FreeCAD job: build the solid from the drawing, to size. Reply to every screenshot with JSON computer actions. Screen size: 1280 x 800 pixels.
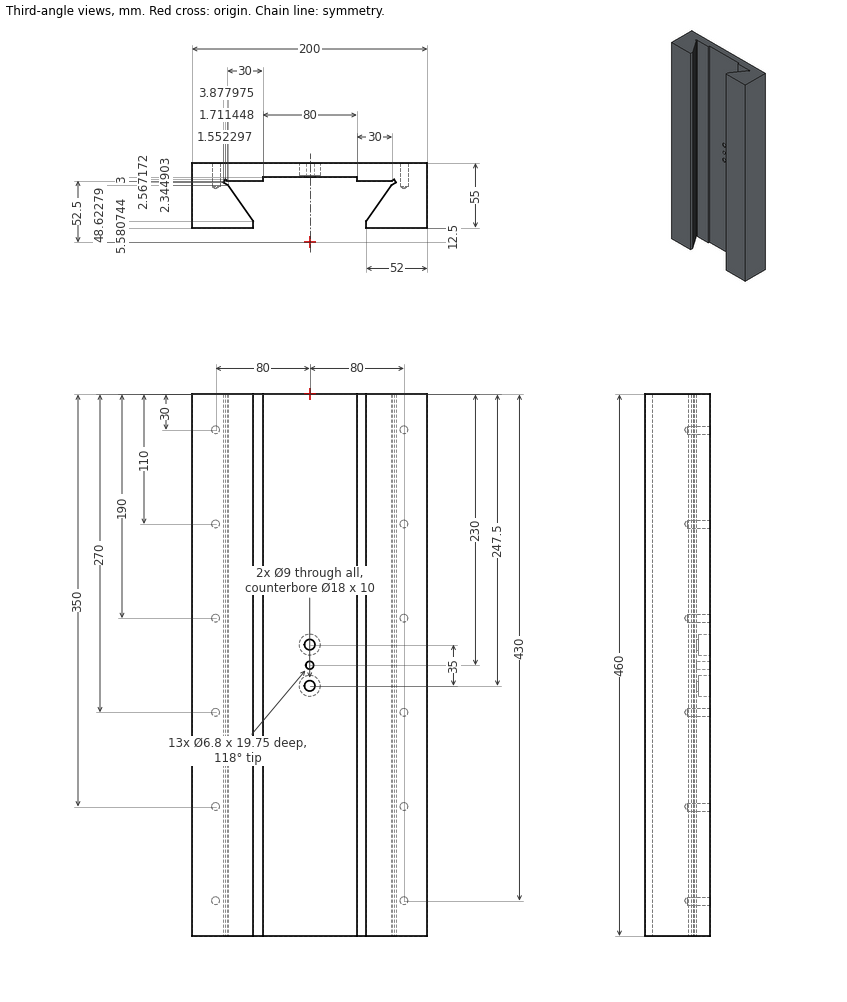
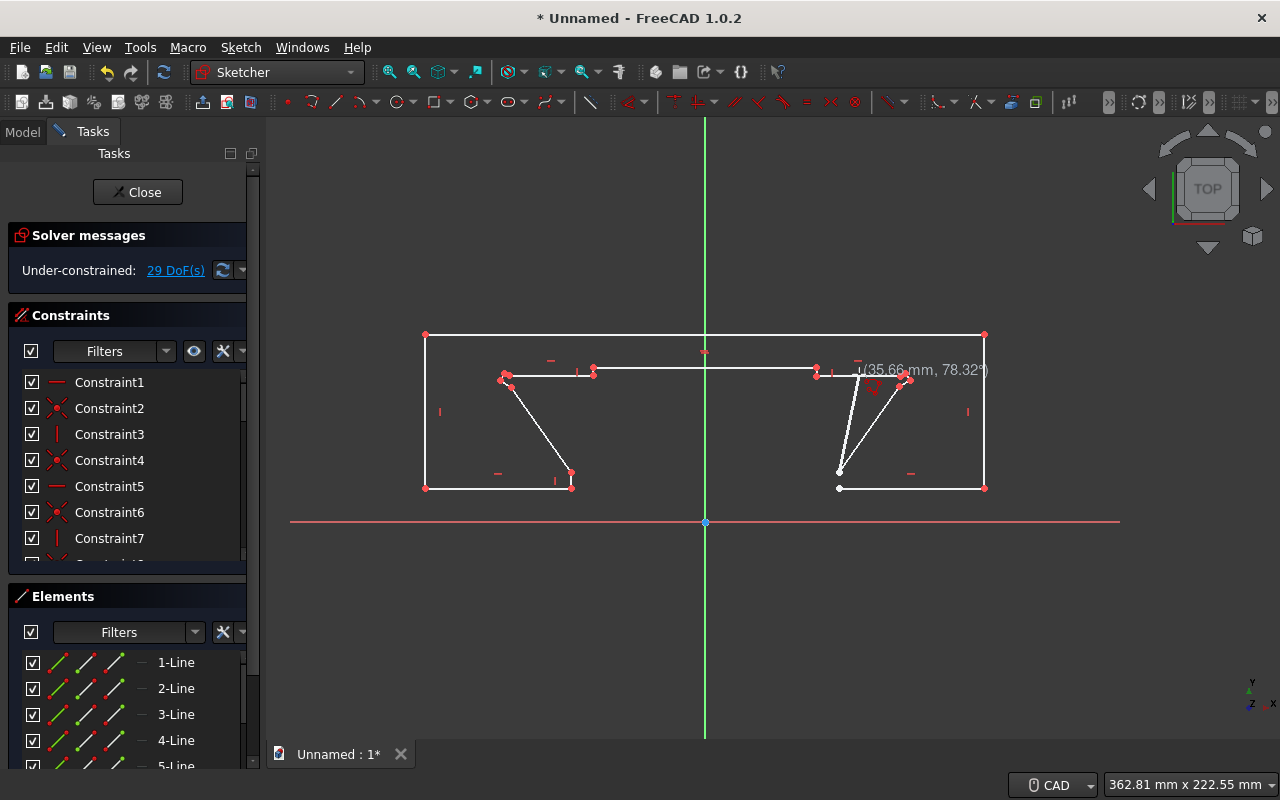
{"action": "left_click", "coordinate": [839, 489]}
{"action": "key", "text": "Escape"}
{"action": "key", "text": "Escape"}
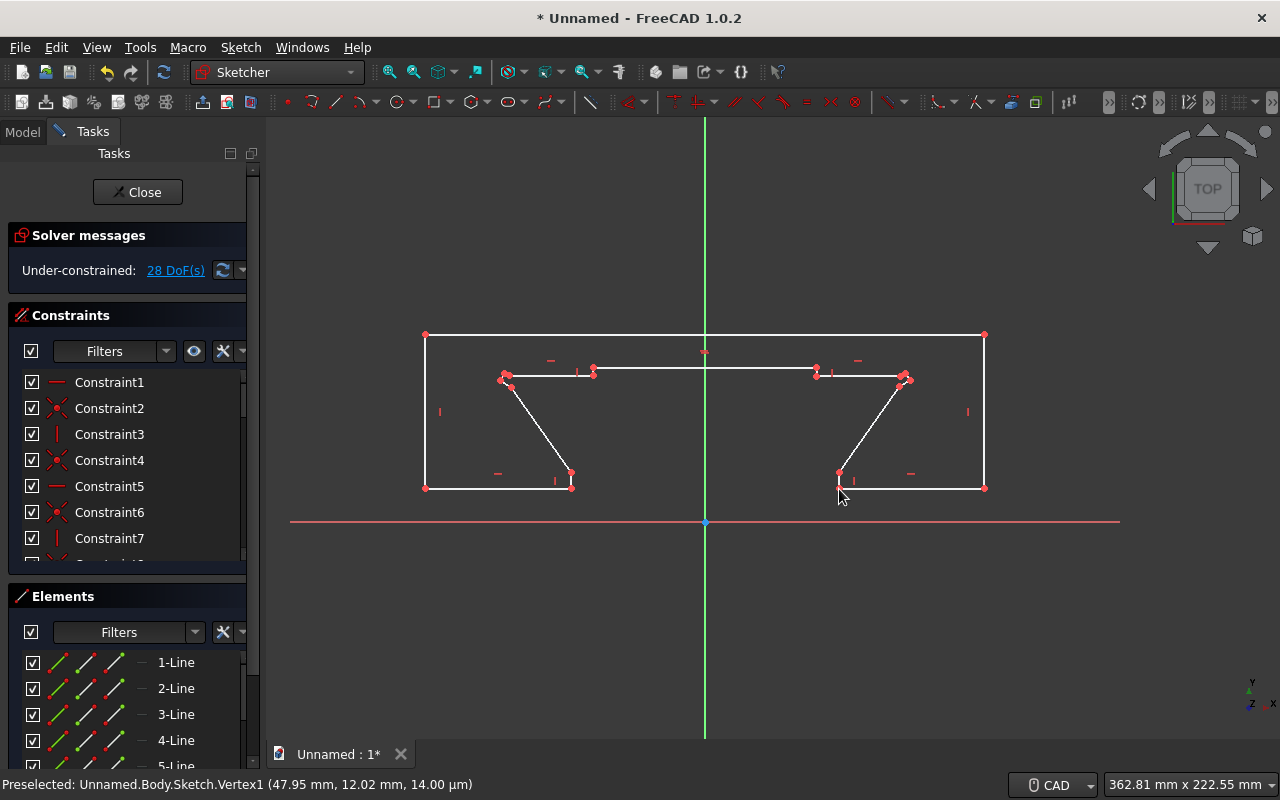
{"action": "left_click", "coordinate": [984, 489]}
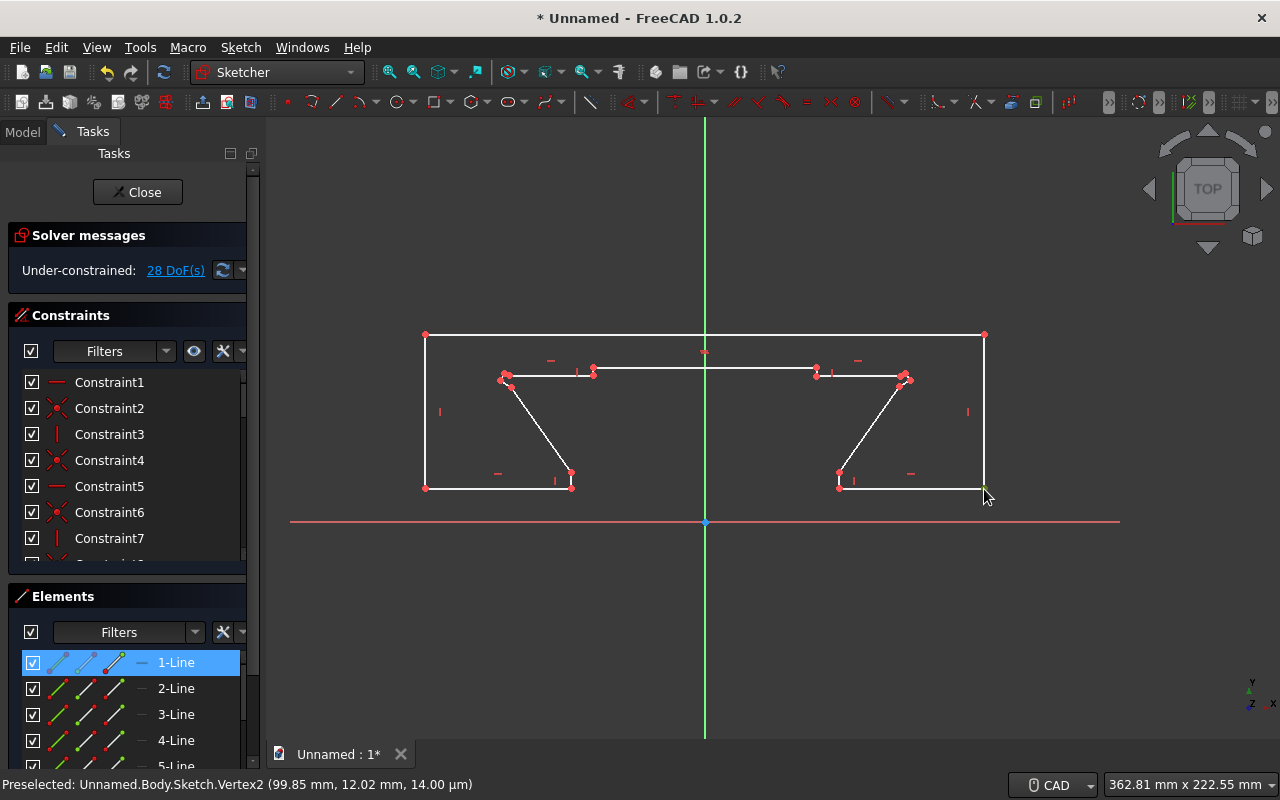
{"action": "left_click", "coordinate": [425, 489]}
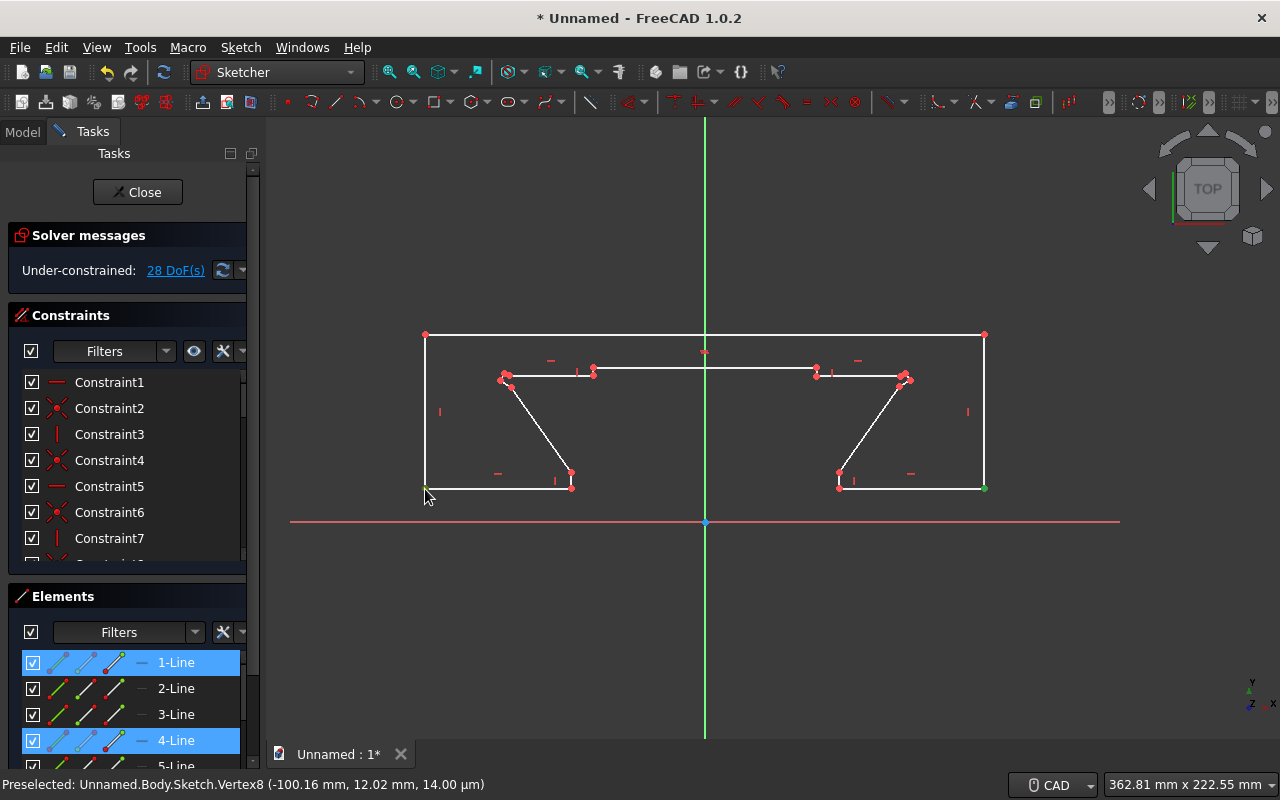
{"action": "left_click", "coordinate": [705, 671]}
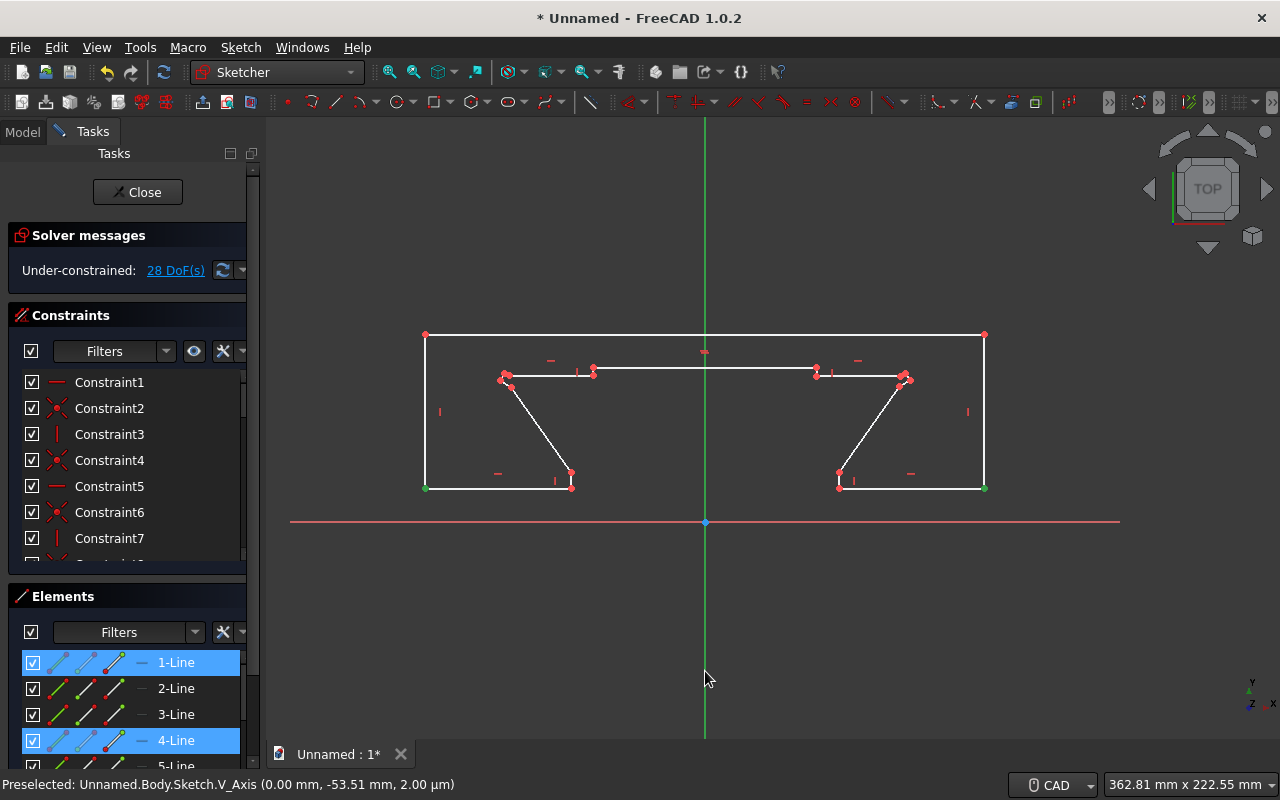
{"action": "left_click", "coordinate": [832, 102]}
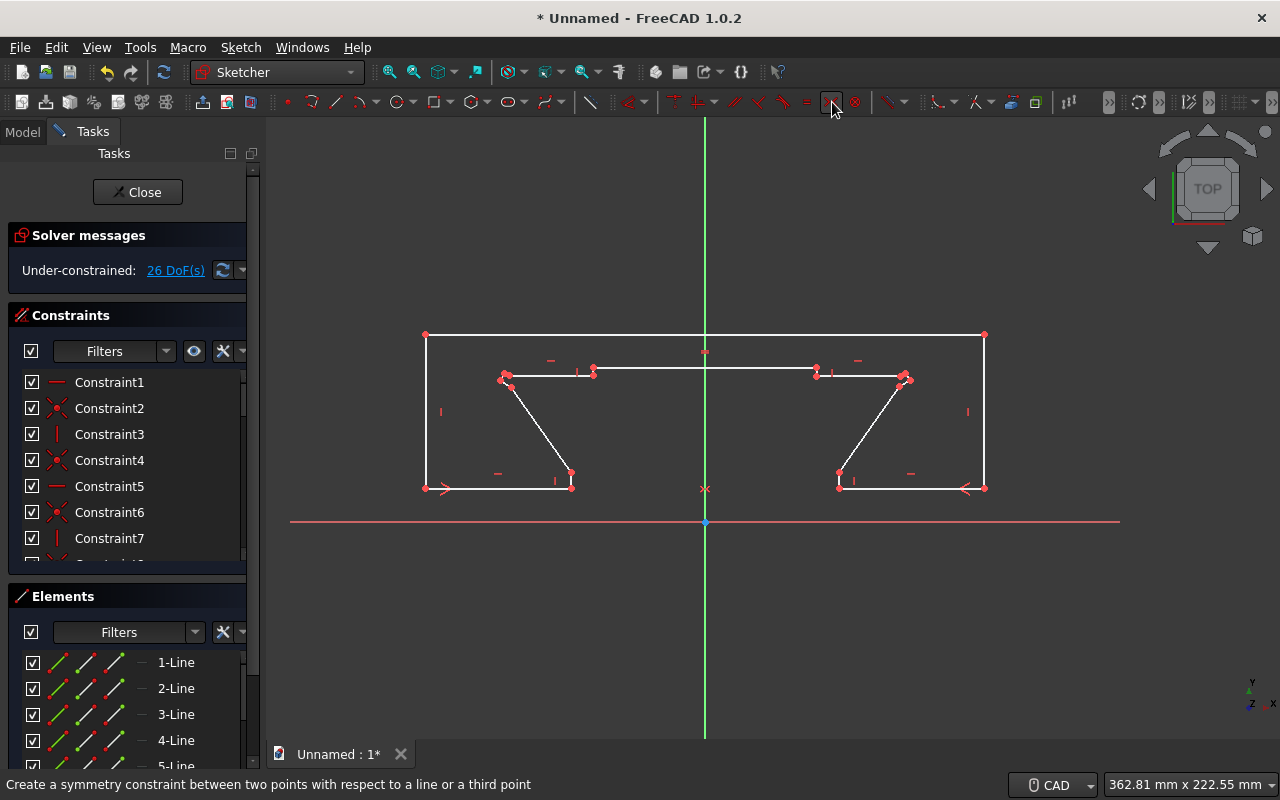
{"action": "scroll", "coordinate": [593, 376], "scroll_direction": "up", "scroll_amount": 3}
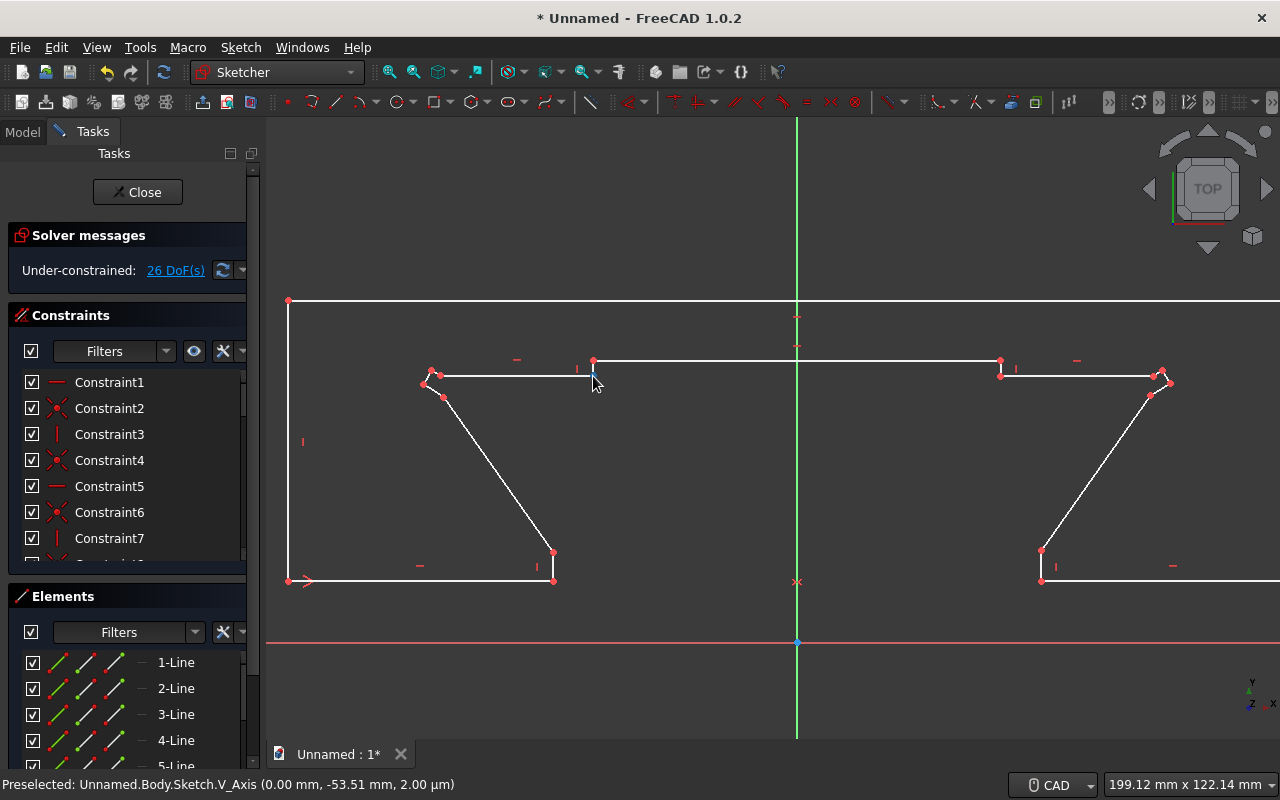
{"action": "left_click", "coordinate": [593, 376]}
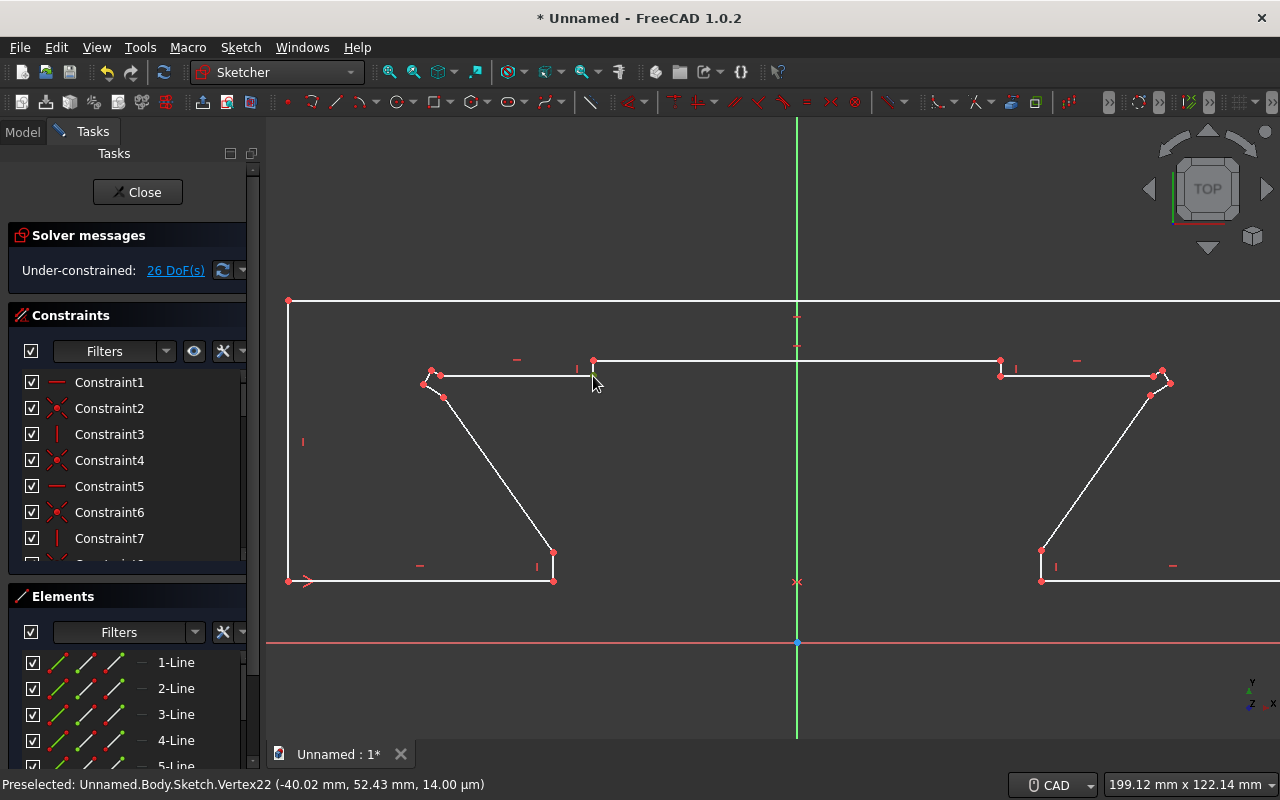
{"action": "left_click", "coordinate": [1001, 376]}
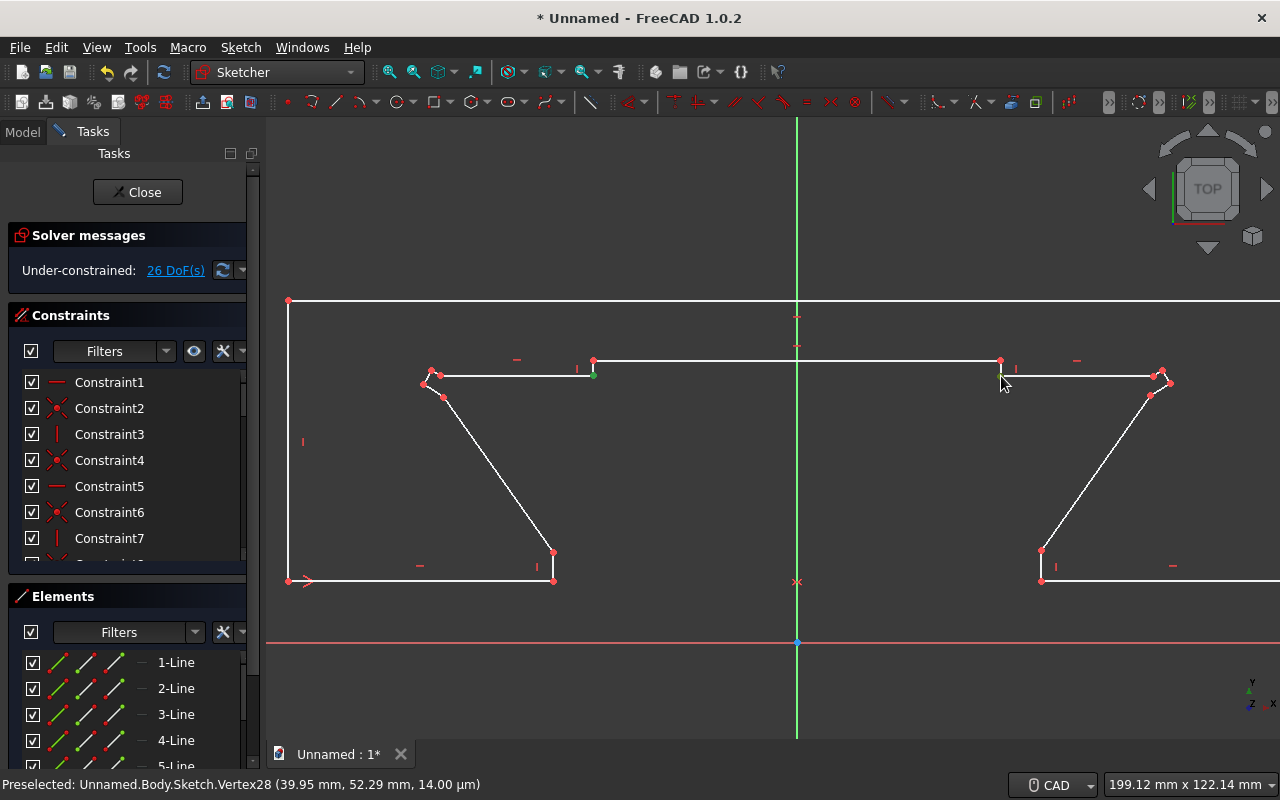
{"action": "left_click", "coordinate": [797, 590]}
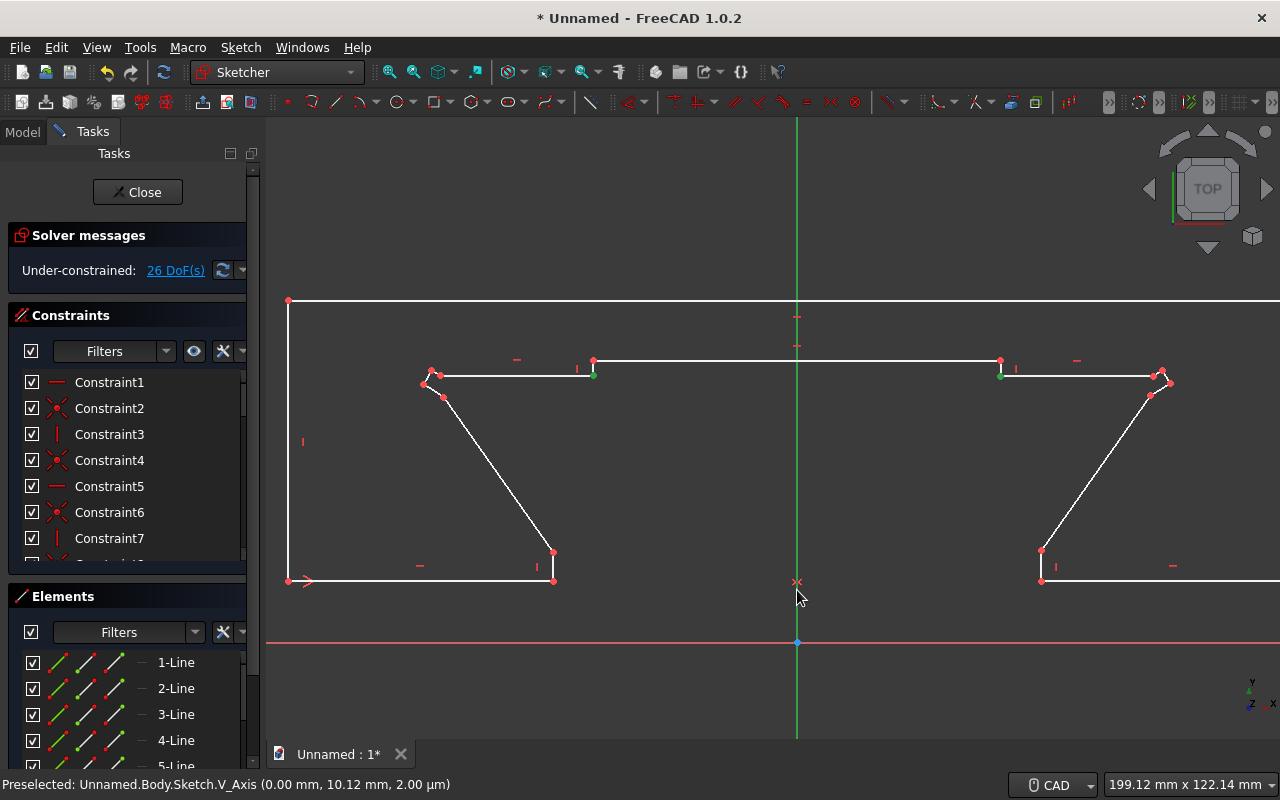
{"action": "left_click", "coordinate": [832, 102]}